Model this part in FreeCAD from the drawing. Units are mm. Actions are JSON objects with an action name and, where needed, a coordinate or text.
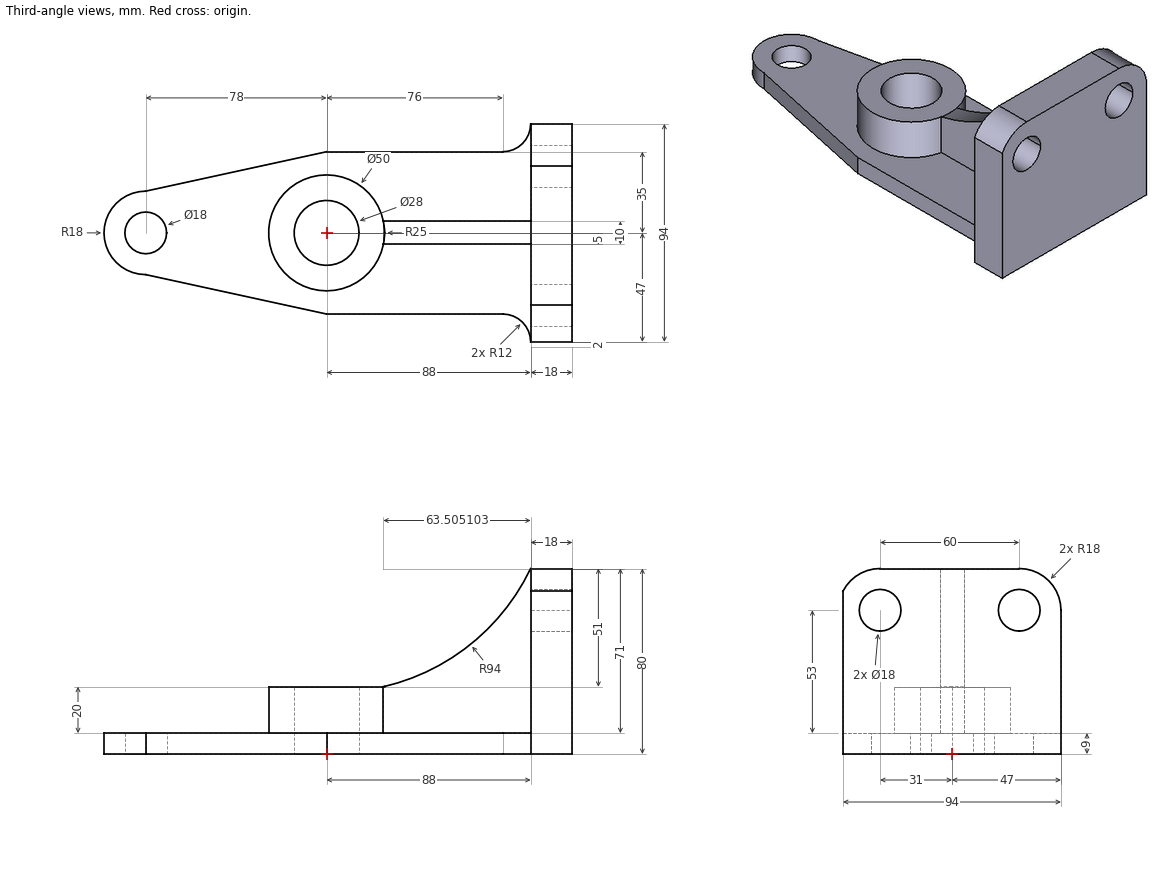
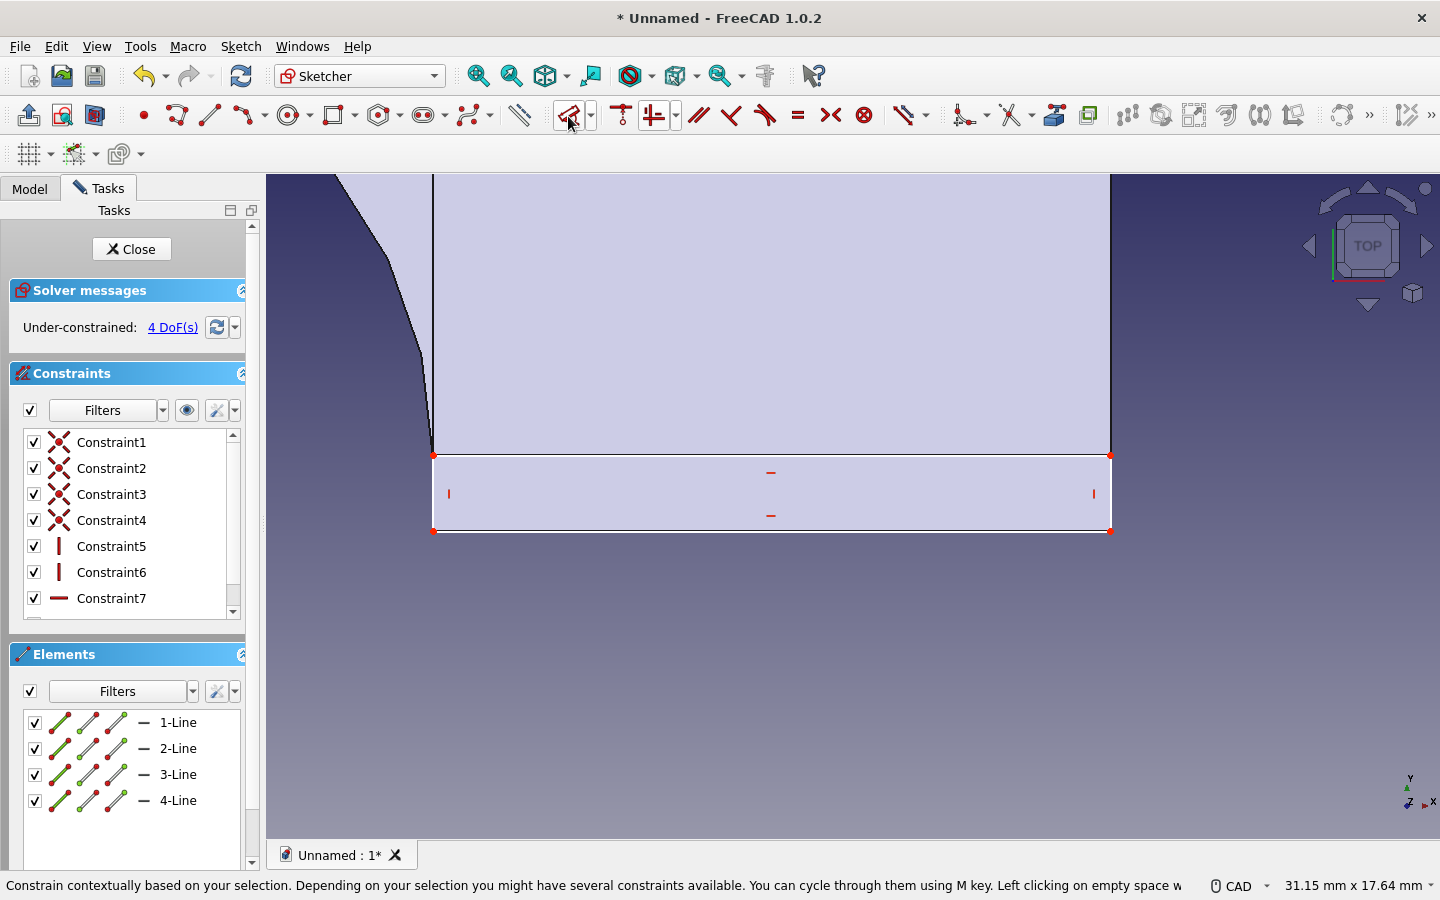
{"action": "left_click", "coordinate": [433, 479]}
{"action": "left_click", "coordinate": [399, 494]}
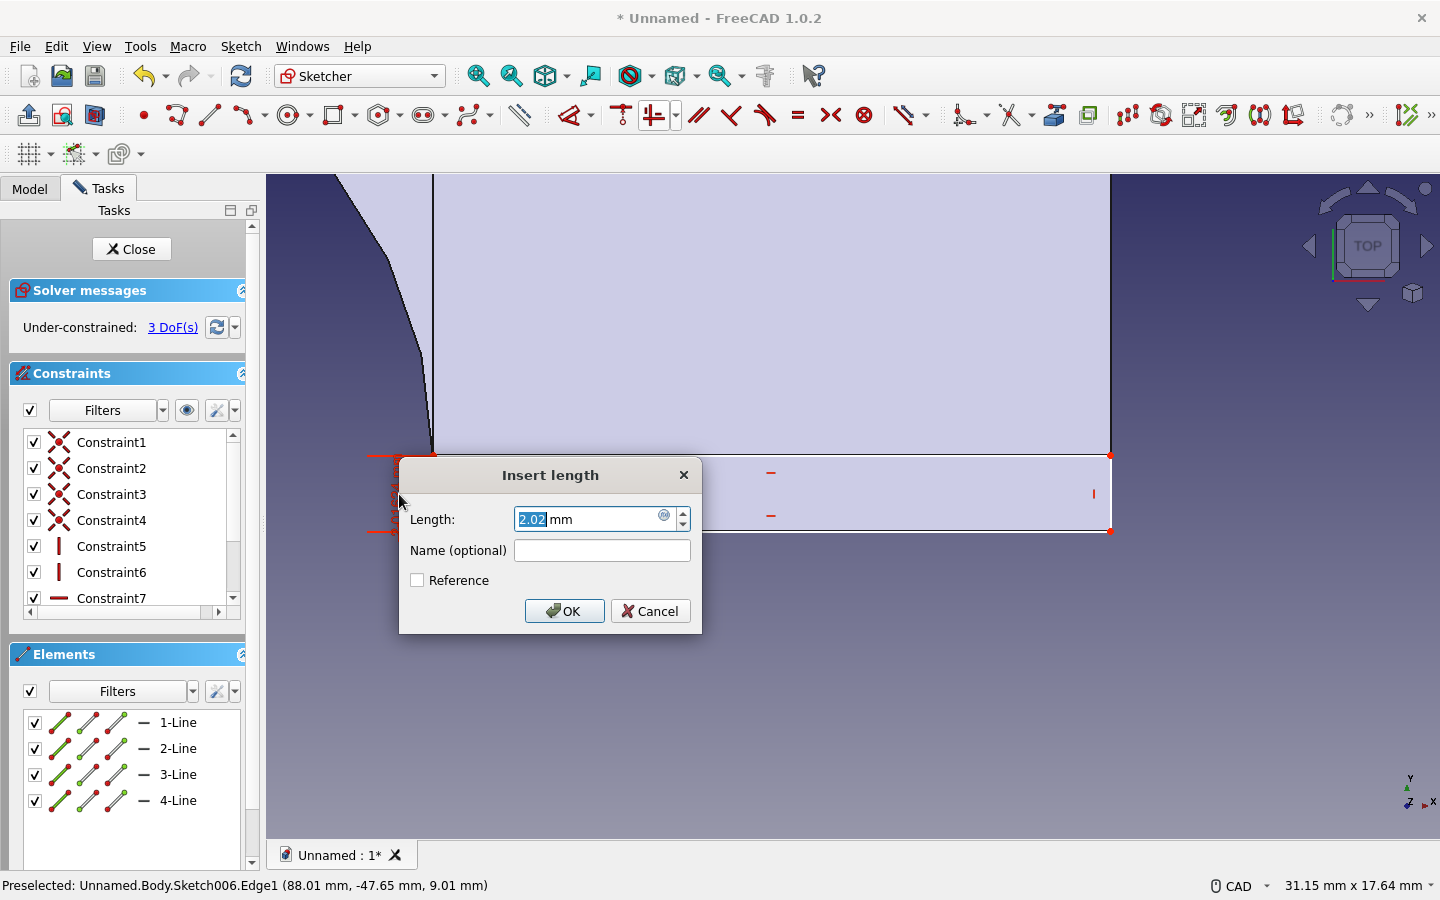
{"action": "type", "text": "2"}
{"action": "key", "text": "Return"}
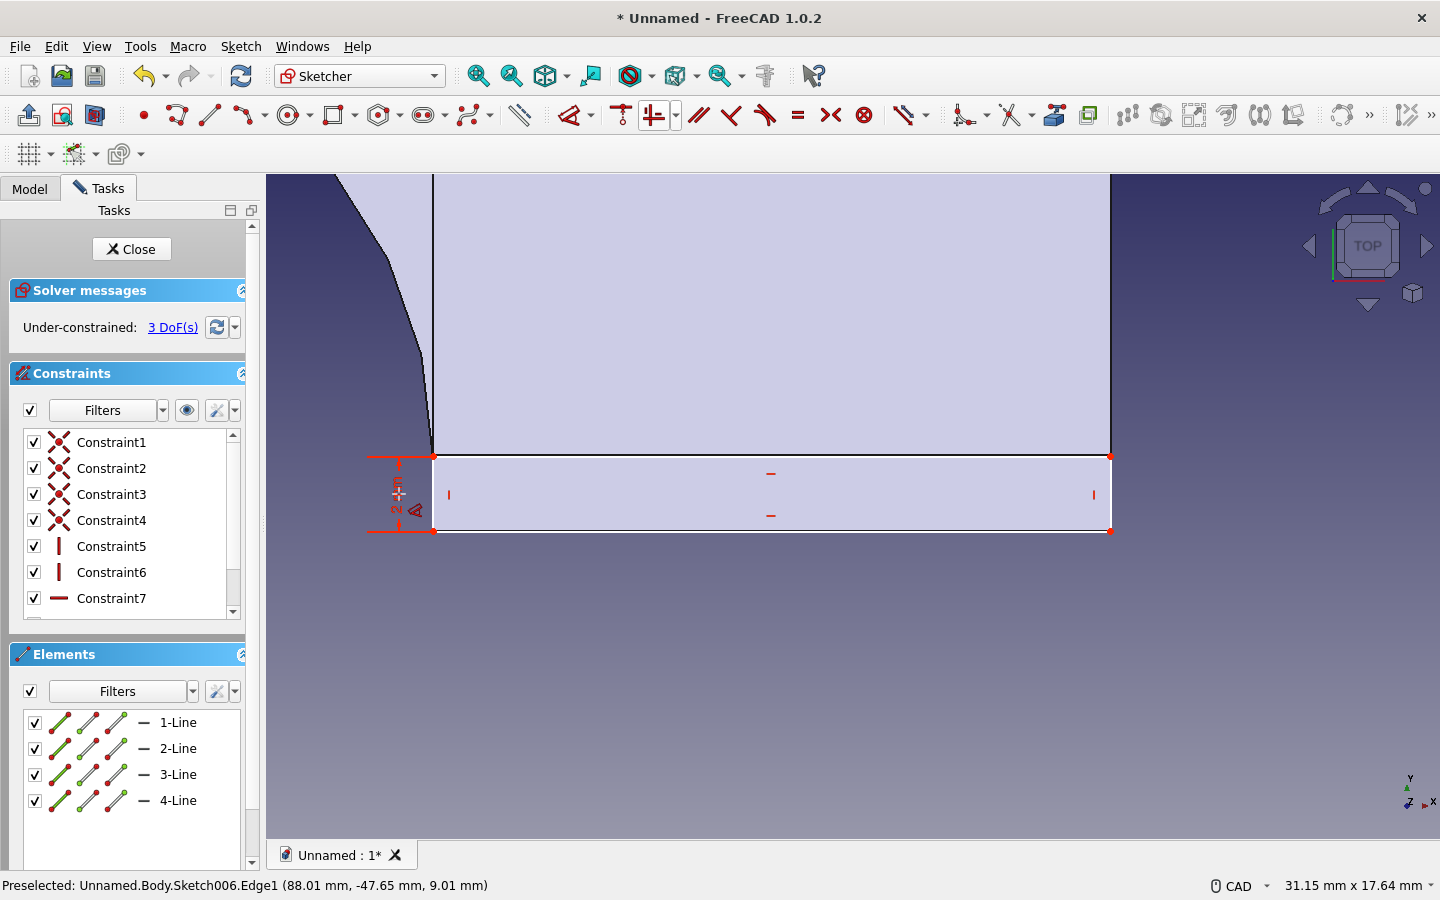
{"action": "left_click", "coordinate": [636, 532]}
{"action": "left_click", "coordinate": [772, 566]}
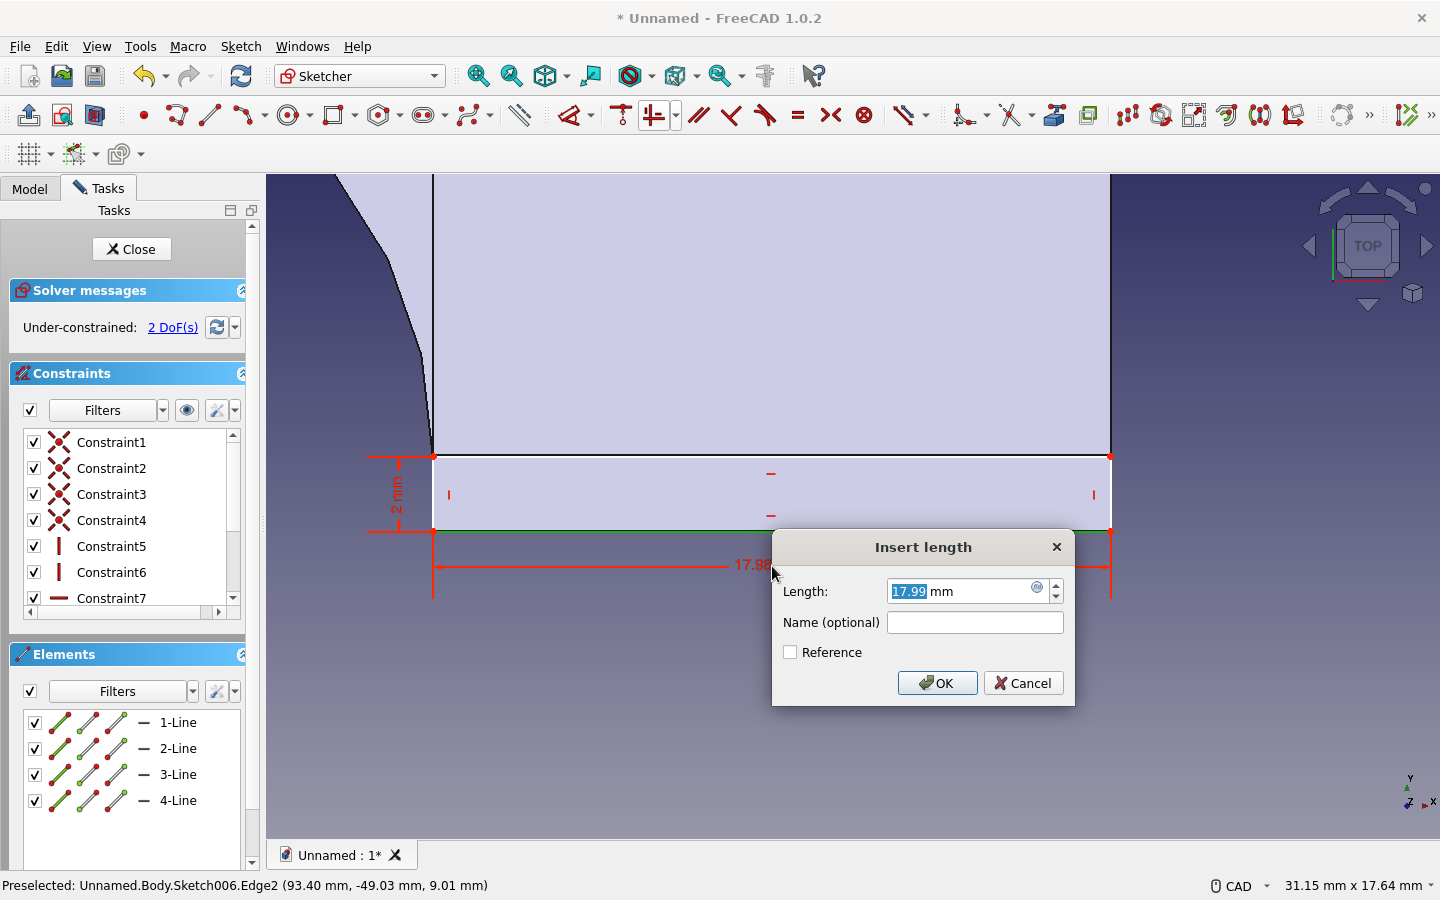
{"action": "type", "text": "18"}
{"action": "key", "text": "Return"}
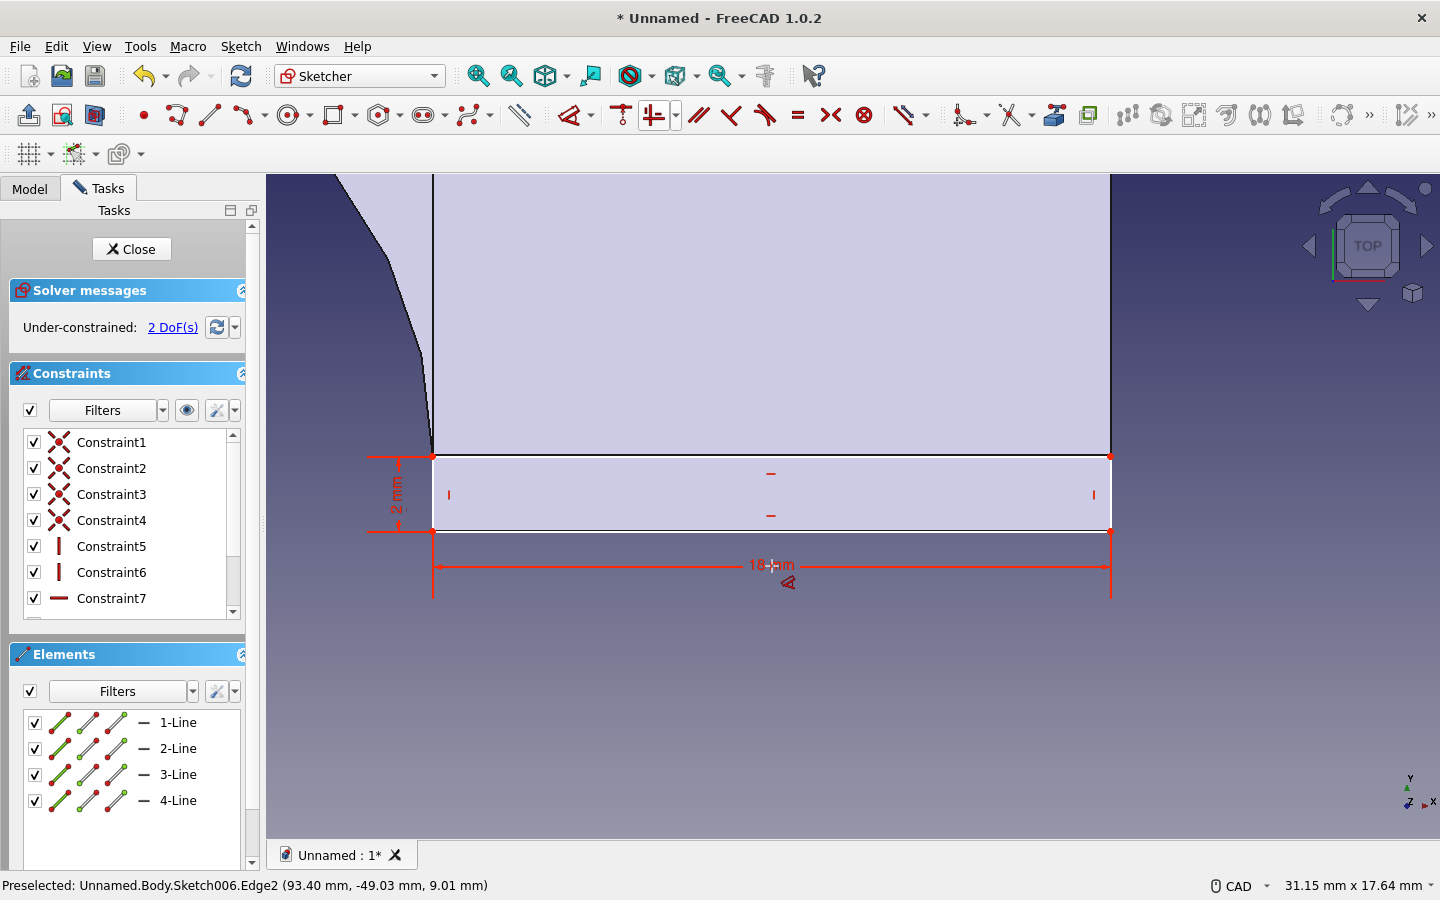
{"action": "left_click", "coordinate": [433, 457]}
{"action": "left_click", "coordinate": [315, 491]}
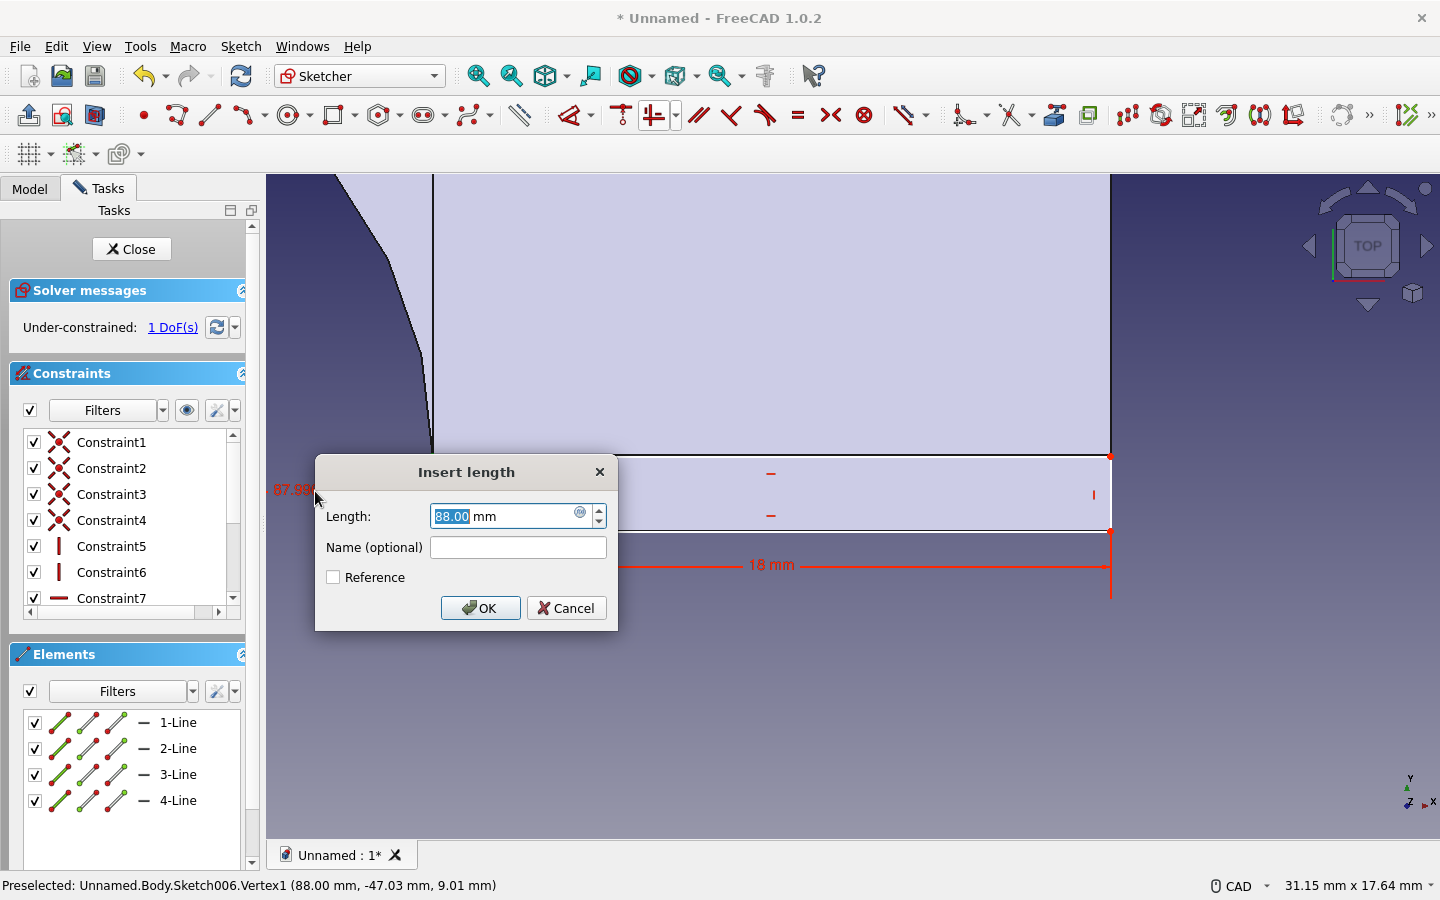
{"action": "type", "text": "88"}
{"action": "key", "text": "Return"}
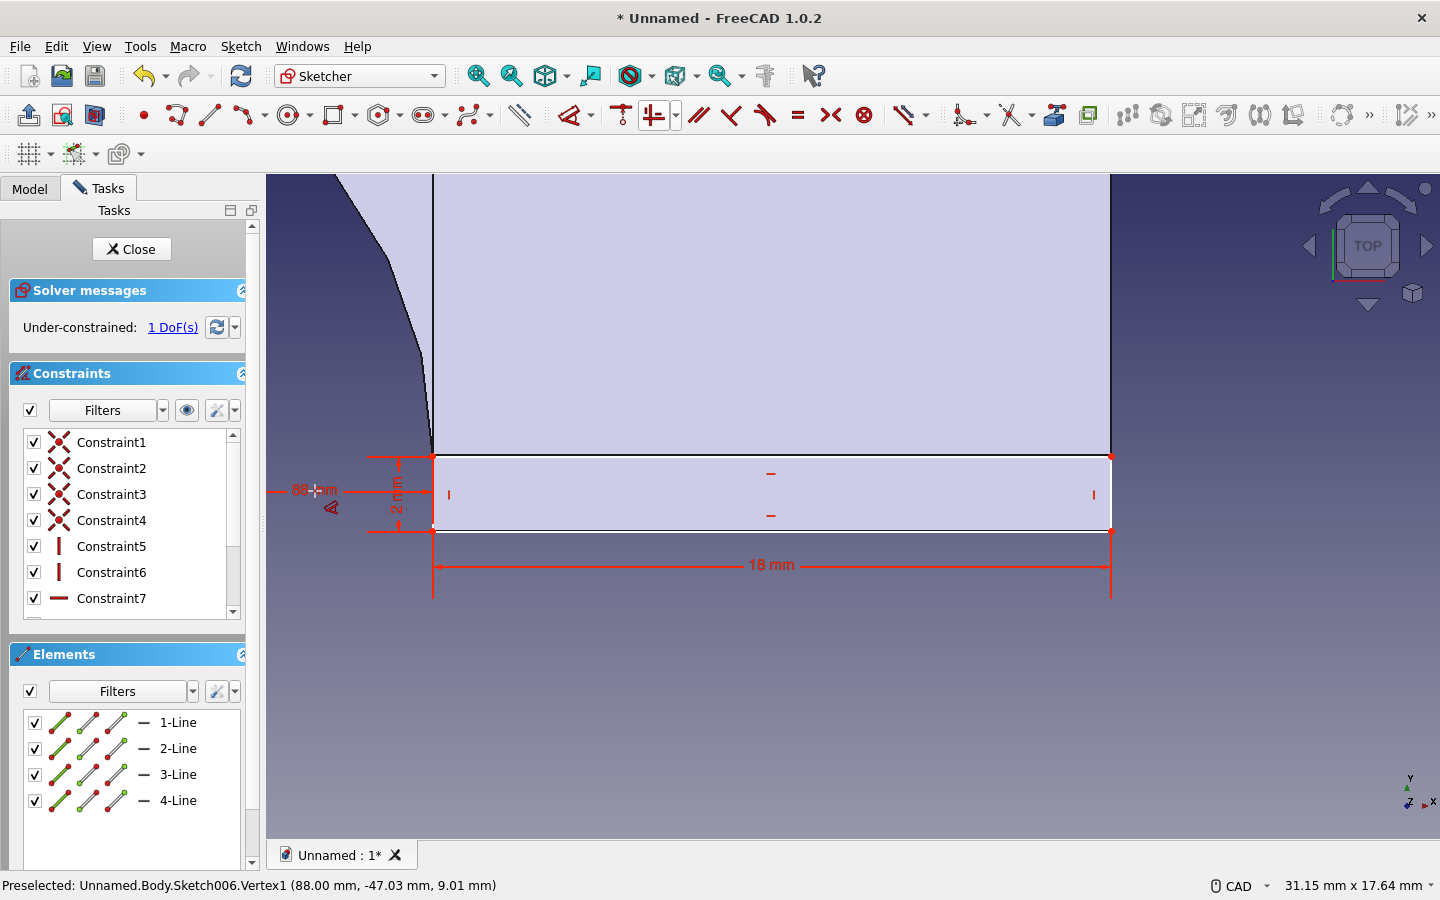
{"action": "left_click", "coordinate": [433, 457]}
{"action": "left_click", "coordinate": [467, 329]}